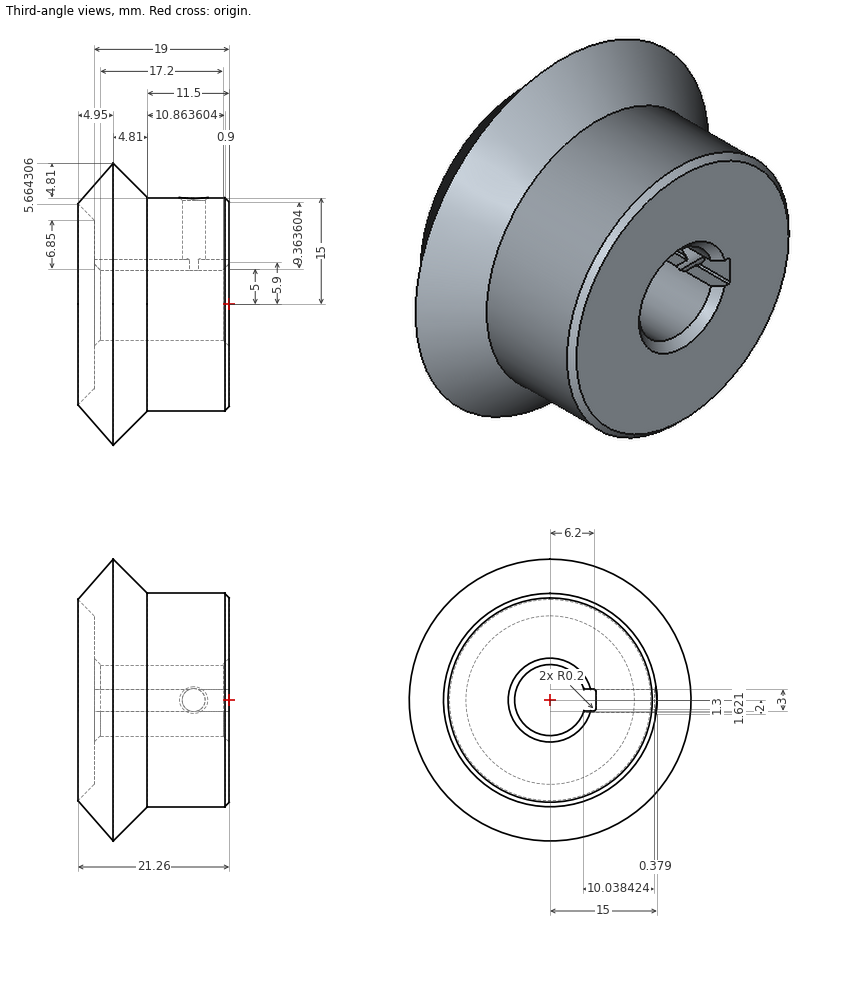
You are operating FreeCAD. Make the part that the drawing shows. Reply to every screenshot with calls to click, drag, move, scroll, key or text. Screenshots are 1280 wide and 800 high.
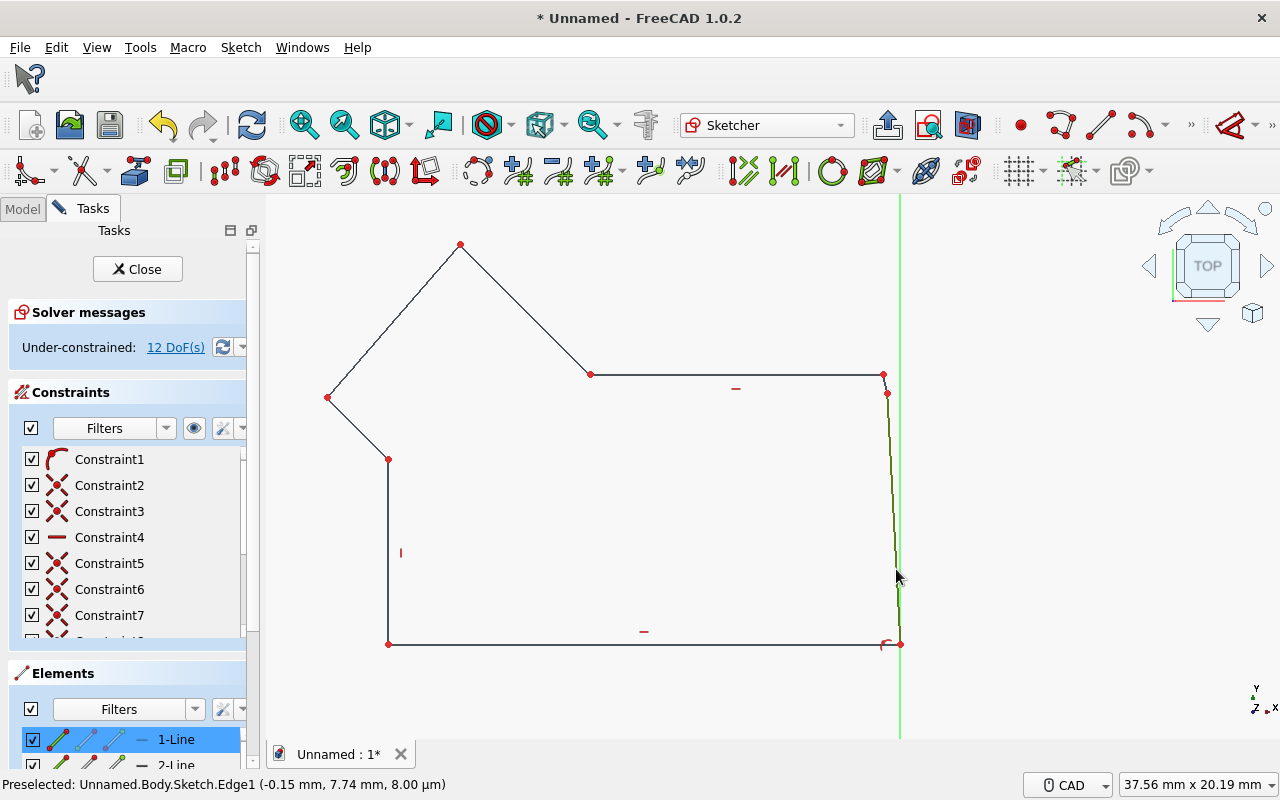
key(v)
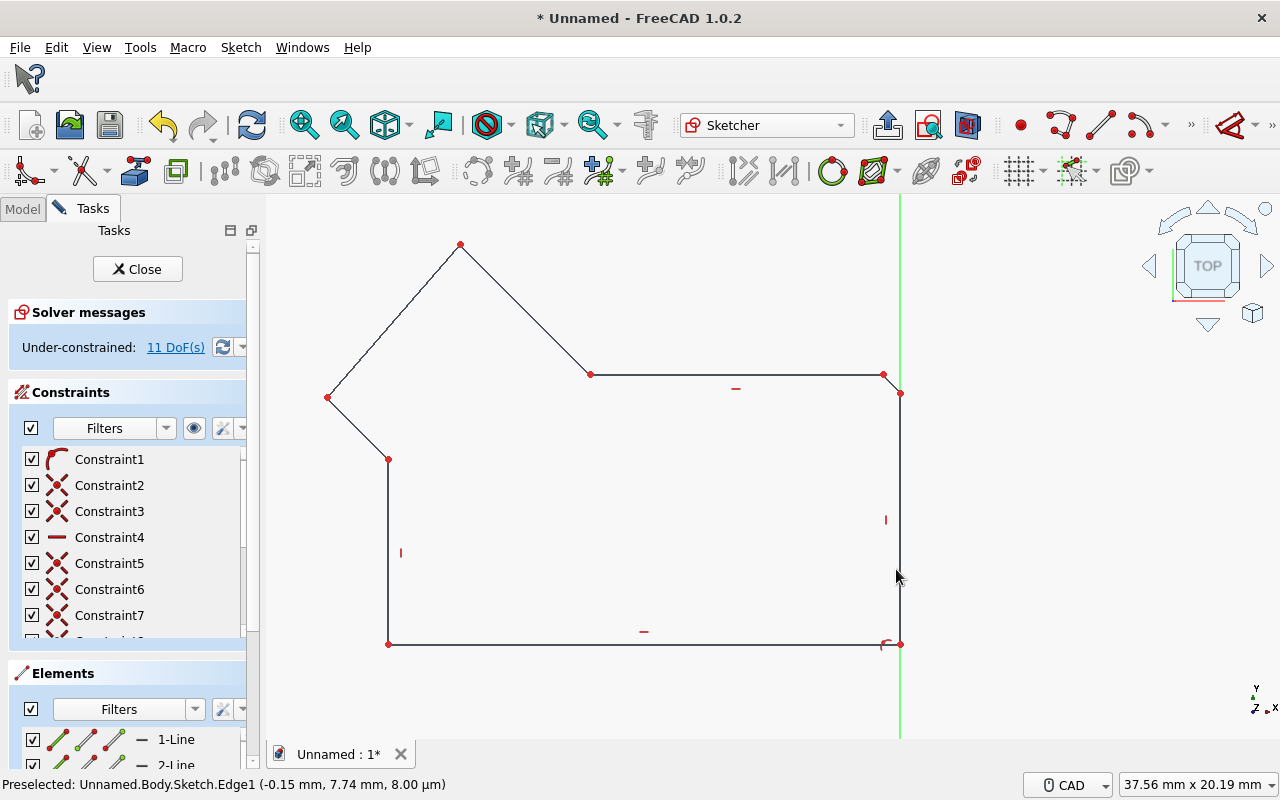
click(542, 645)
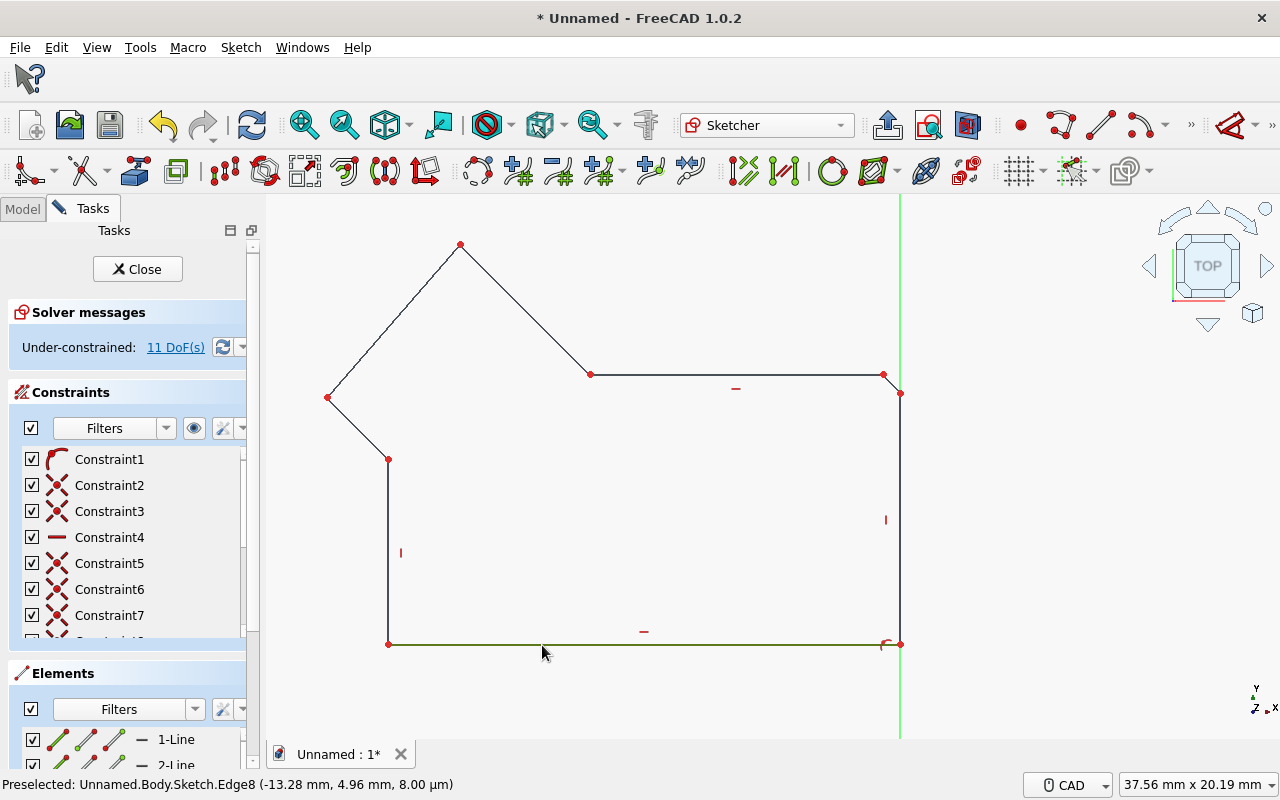
key(l)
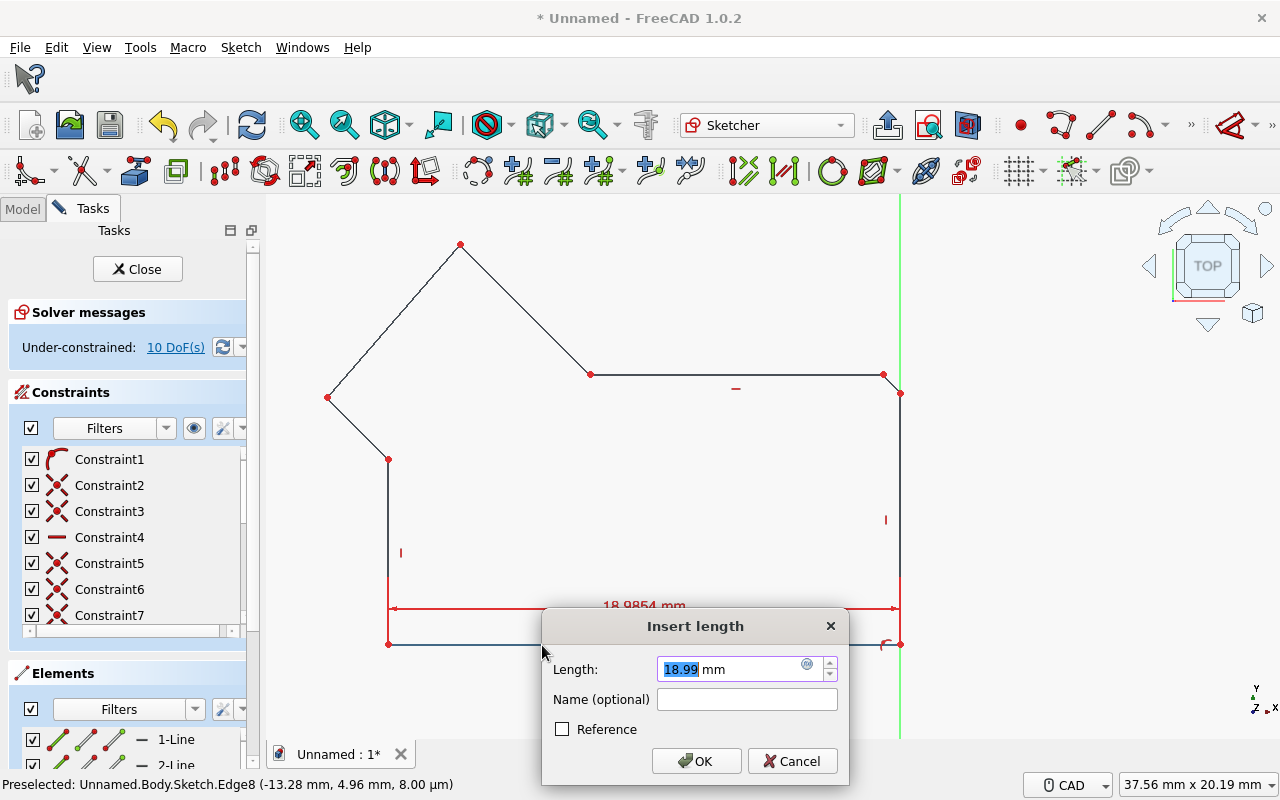
text(19)
key(Return)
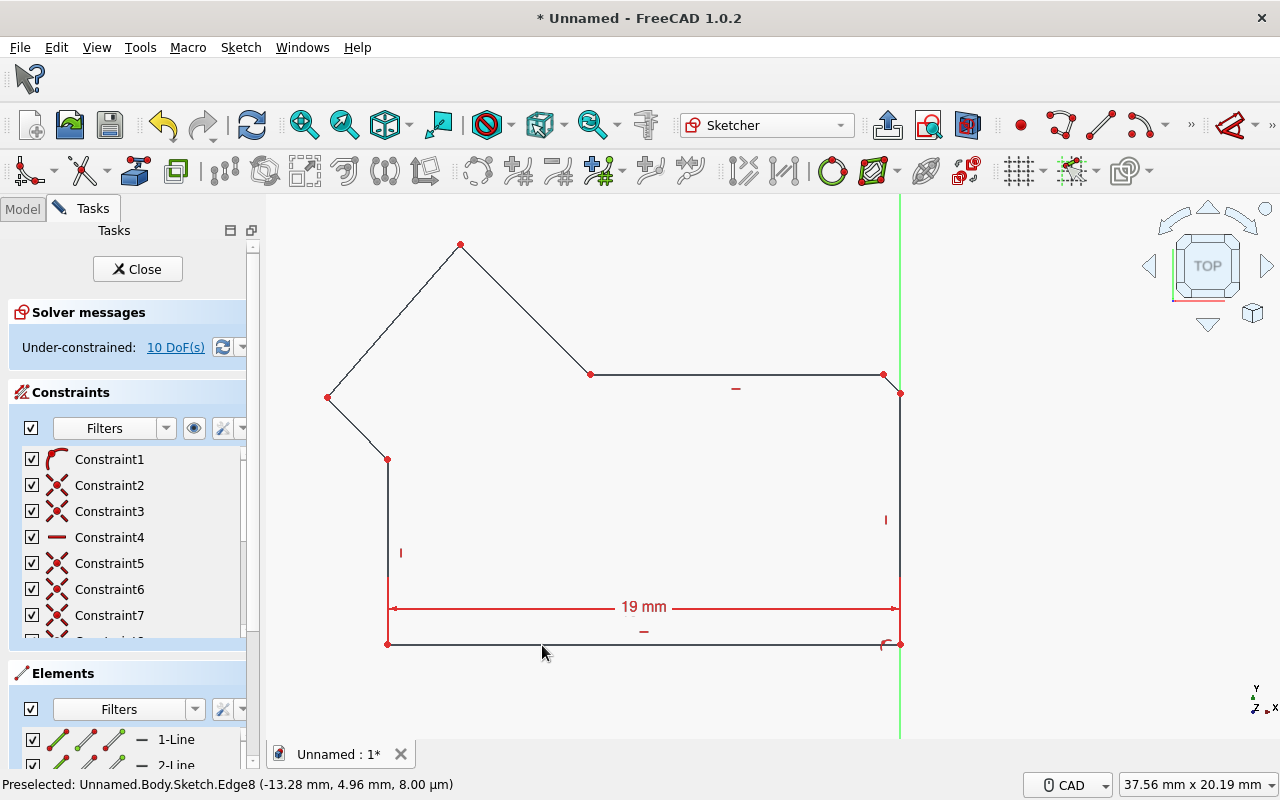
click(900, 645)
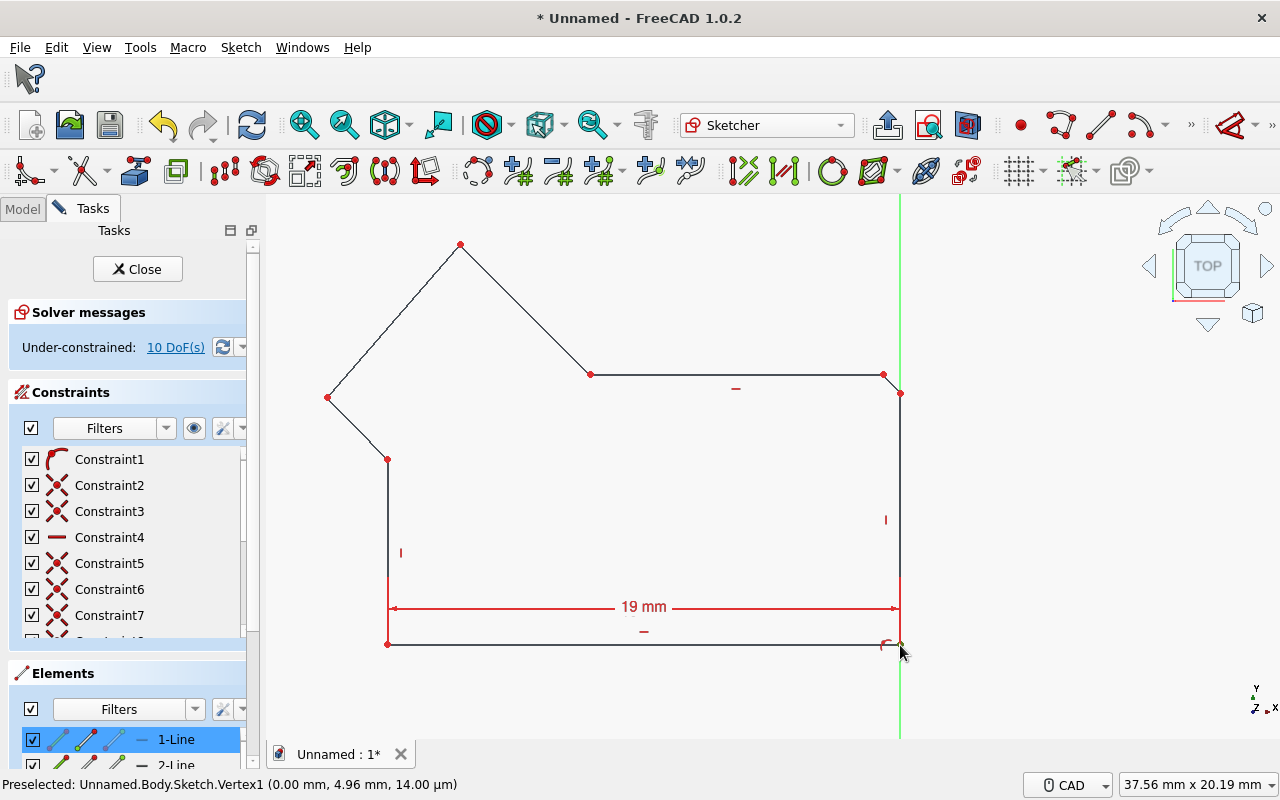
click(1258, 126)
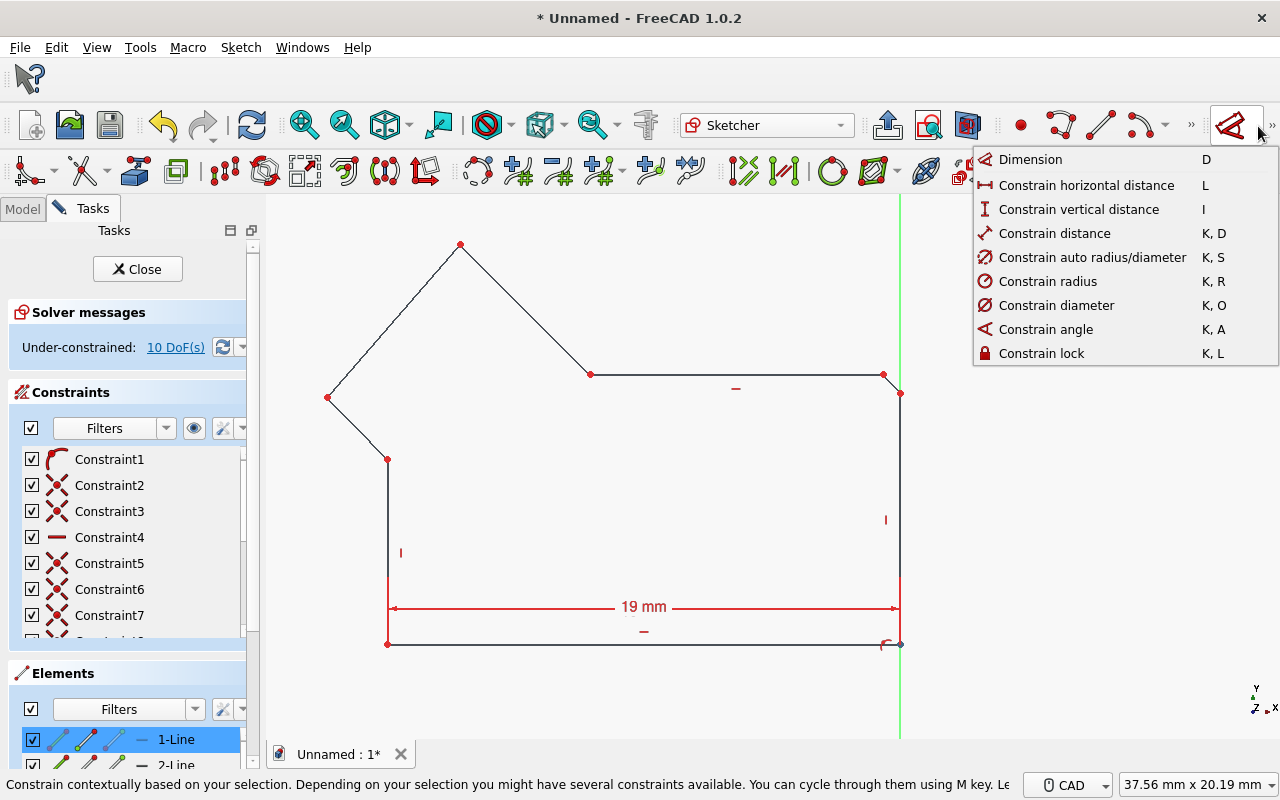
click(1126, 209)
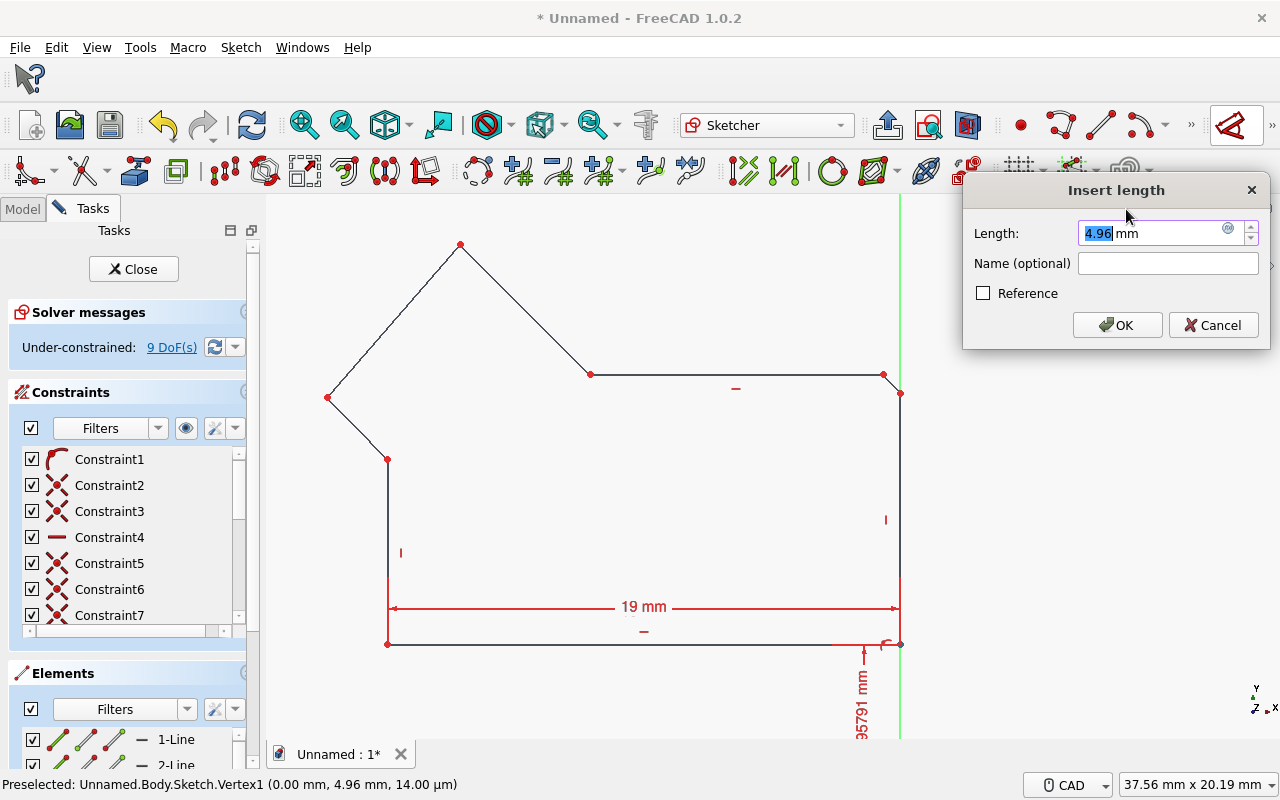
text(5)
key(Return)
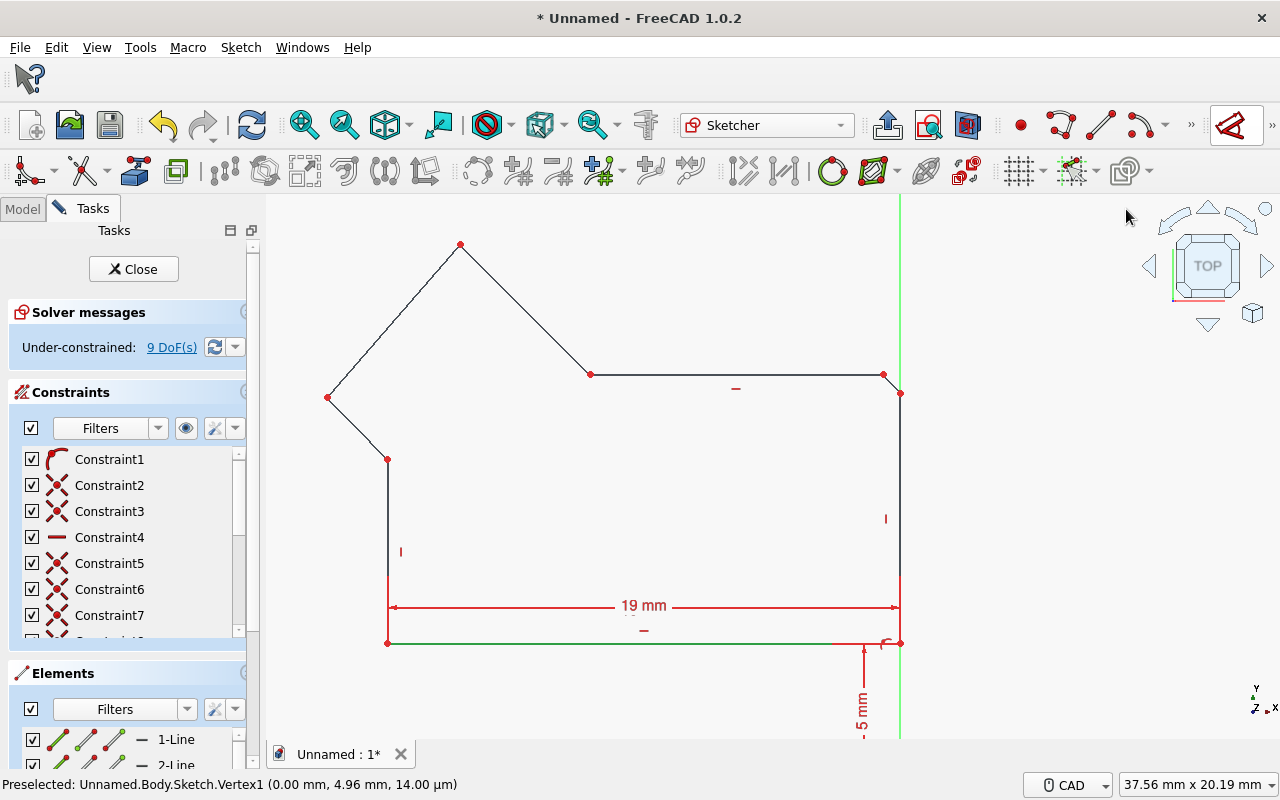
click(883, 375)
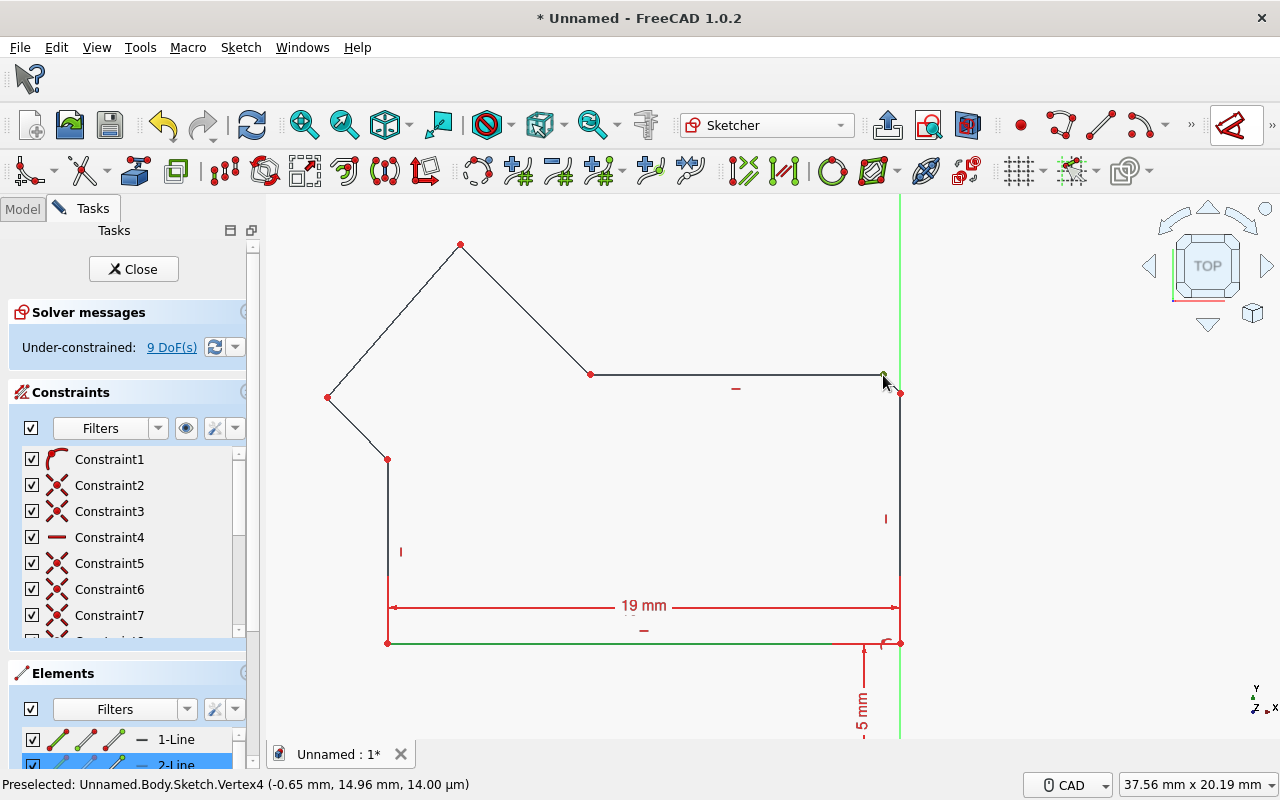
click(1258, 126)